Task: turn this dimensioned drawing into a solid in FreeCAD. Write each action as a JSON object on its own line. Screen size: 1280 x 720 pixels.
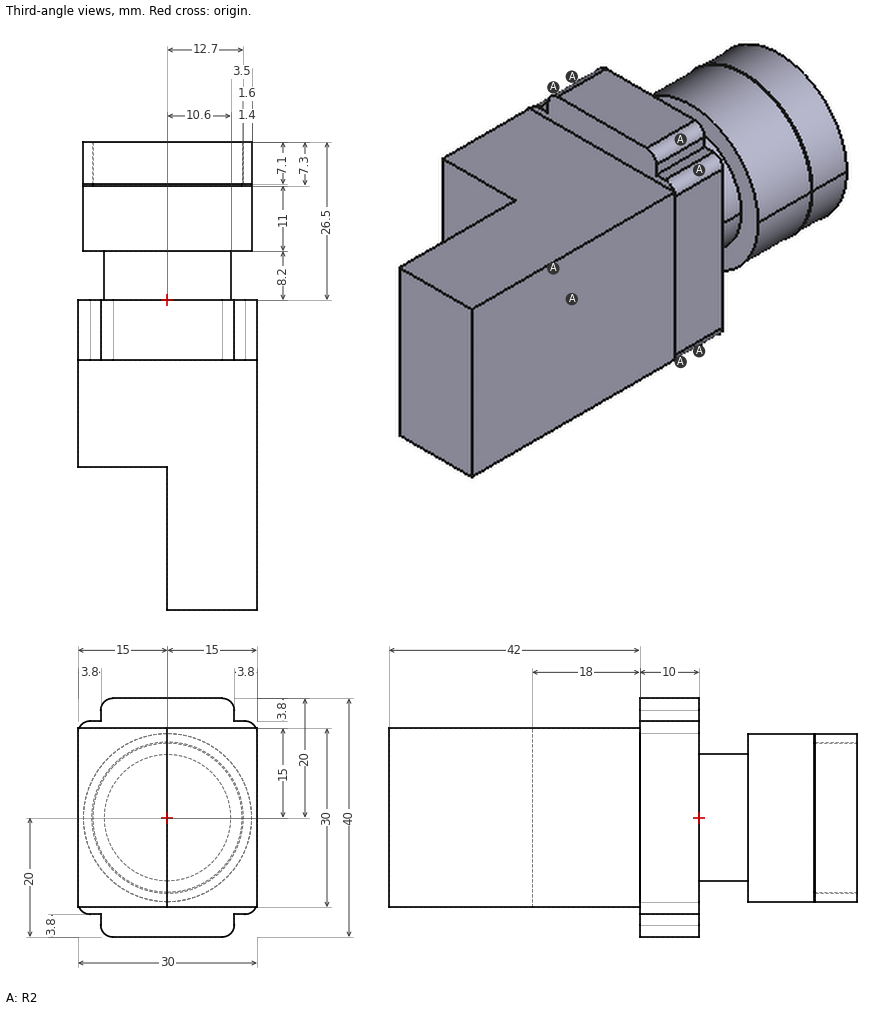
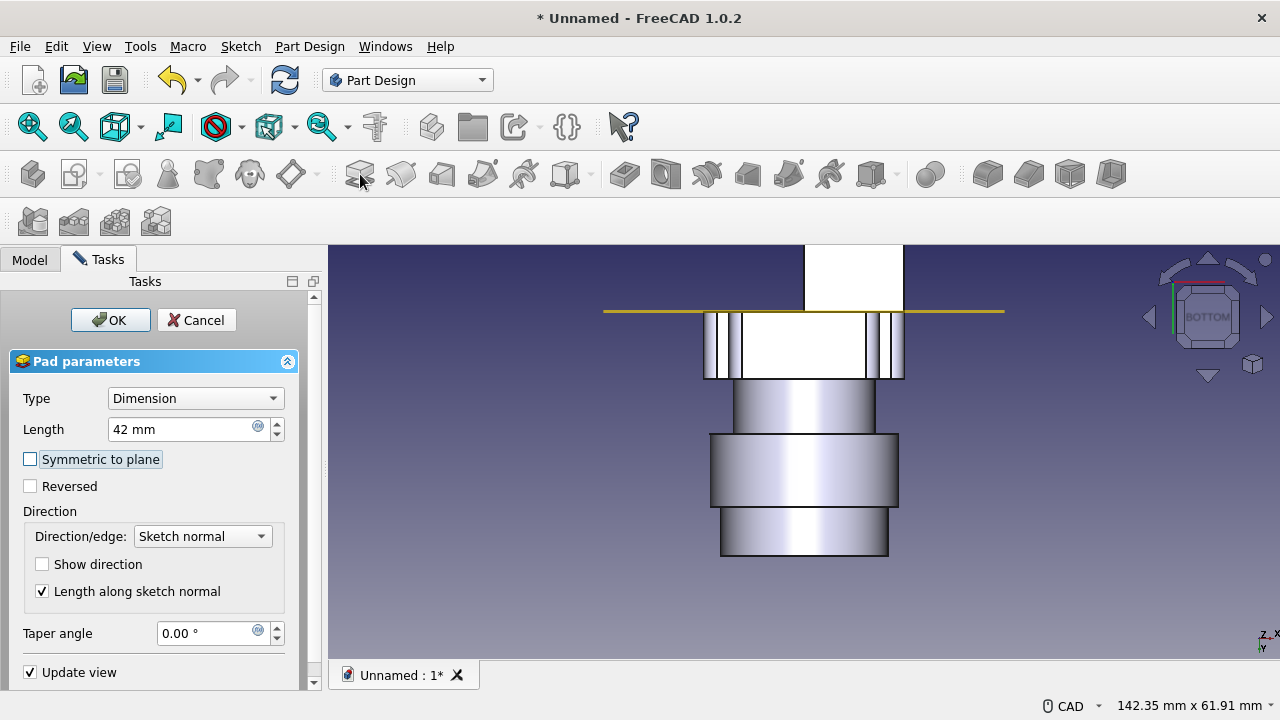
{"action": "left_click", "coordinate": [111, 320]}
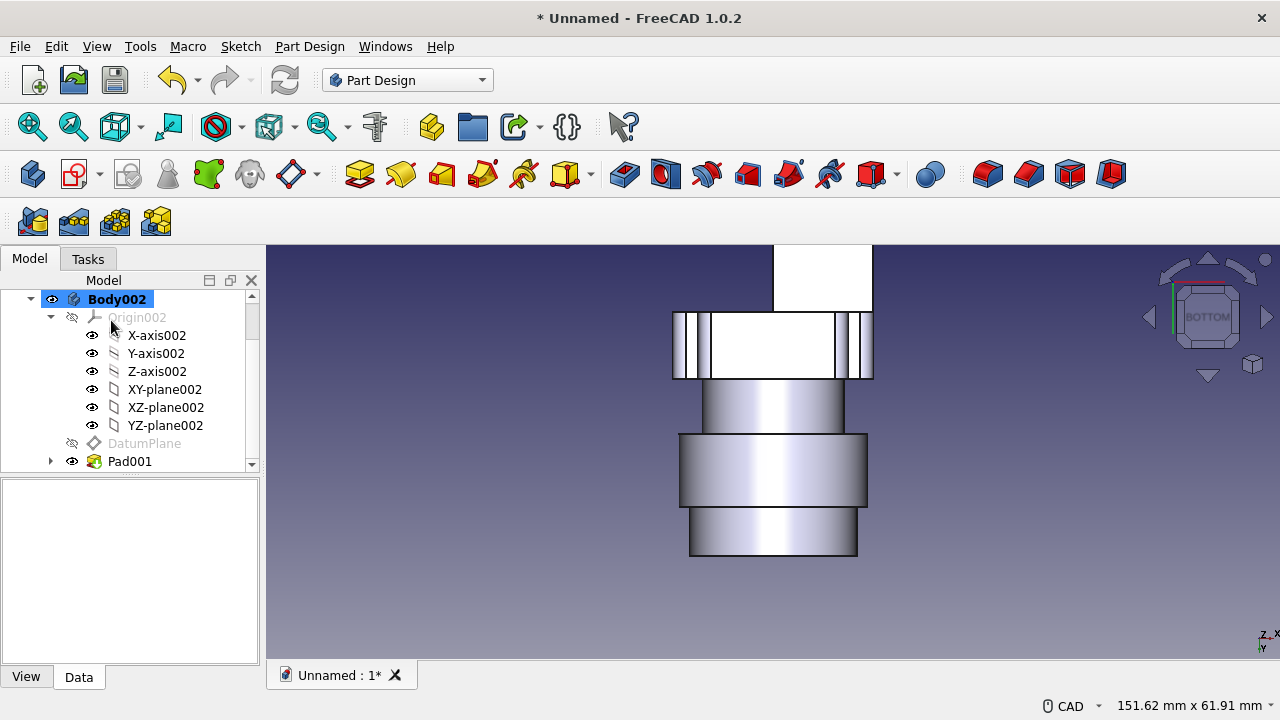
{"action": "key", "text": "v f"}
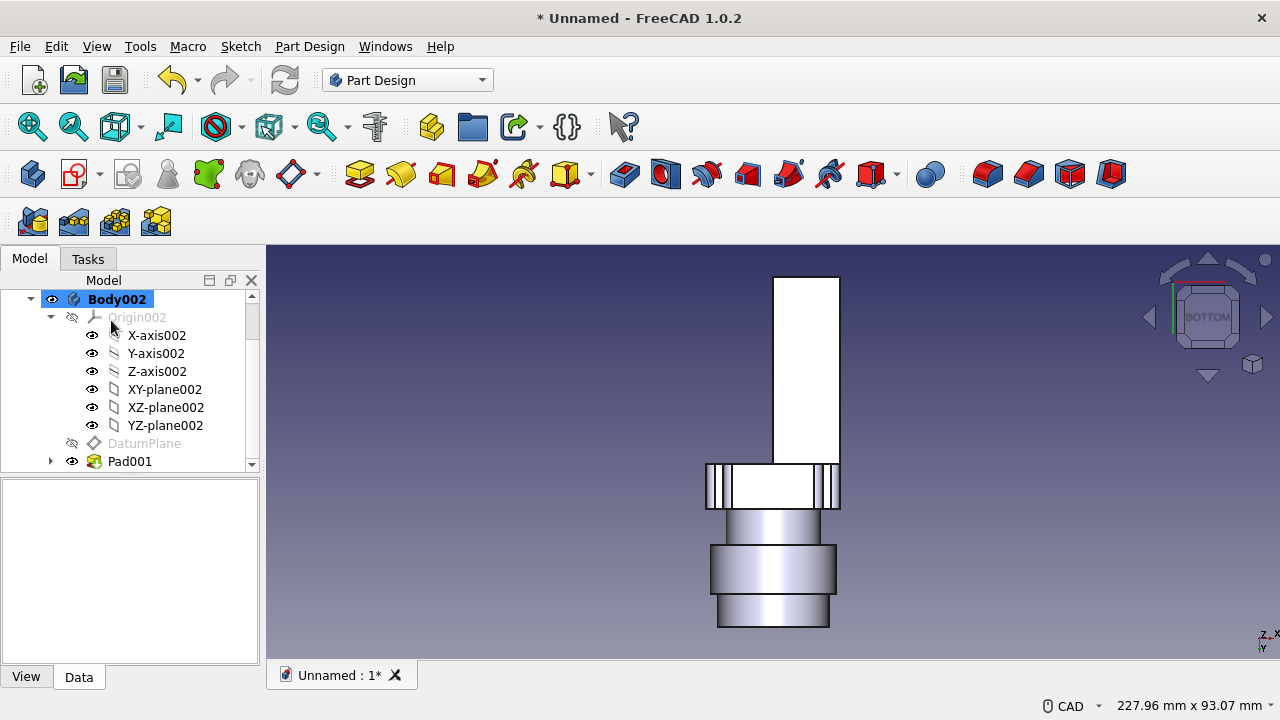
{"action": "key", "text": "4"}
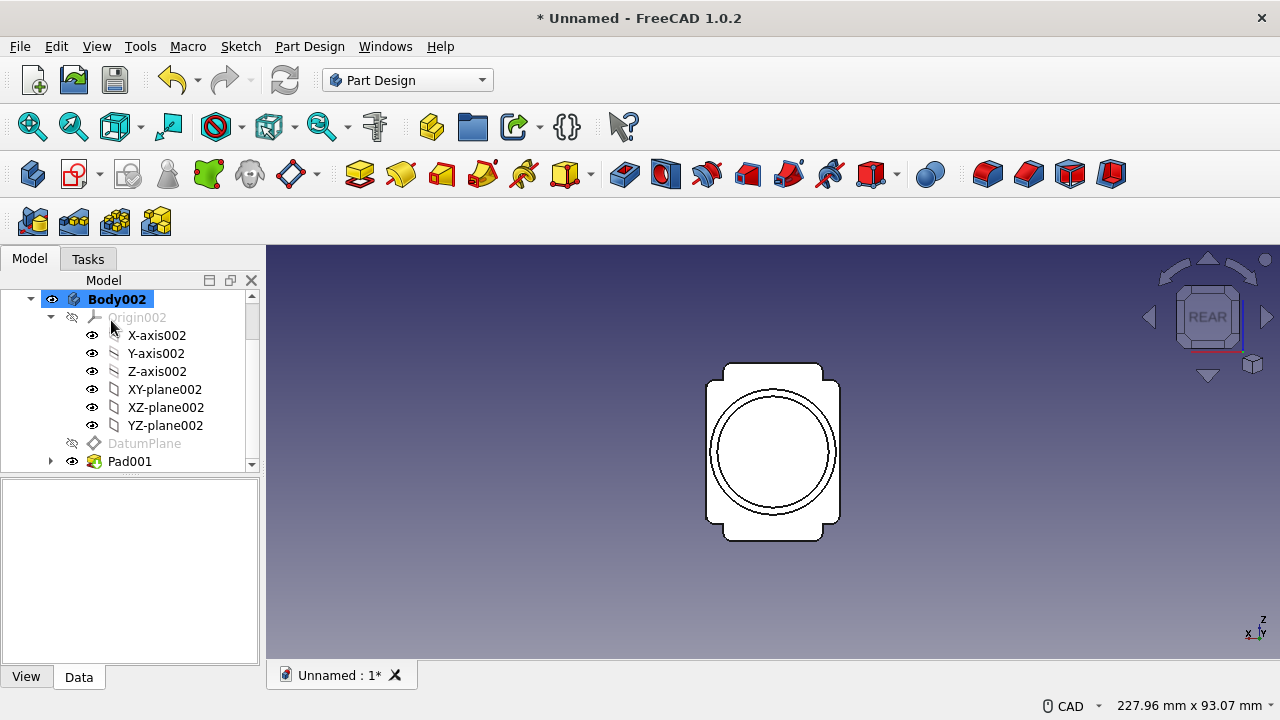
{"action": "key", "text": "v f"}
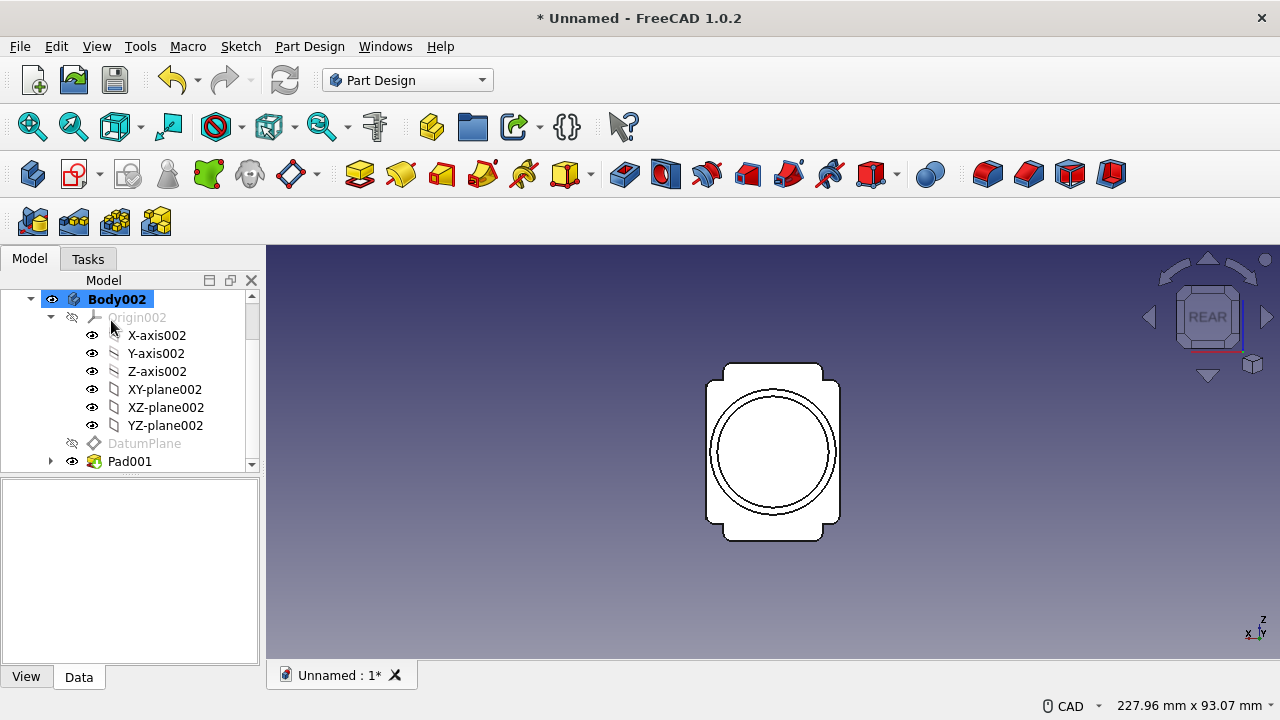
{"action": "key", "text": "5"}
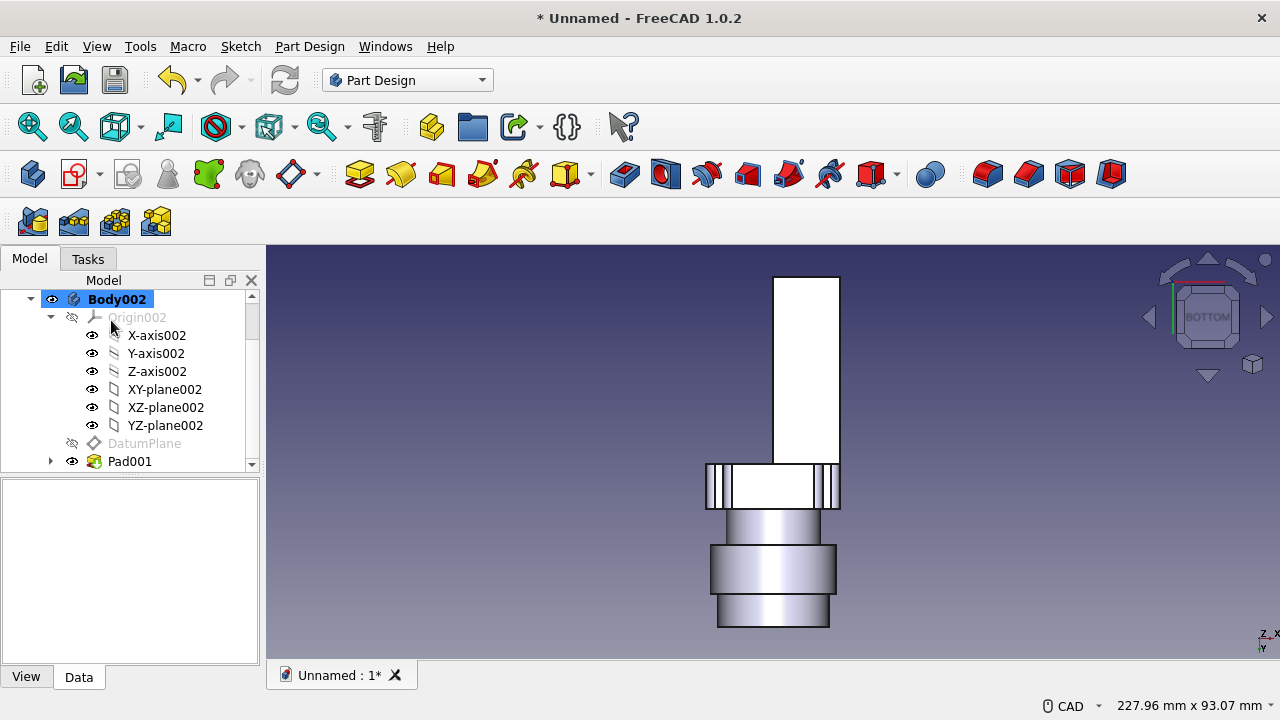
{"action": "key", "text": "3"}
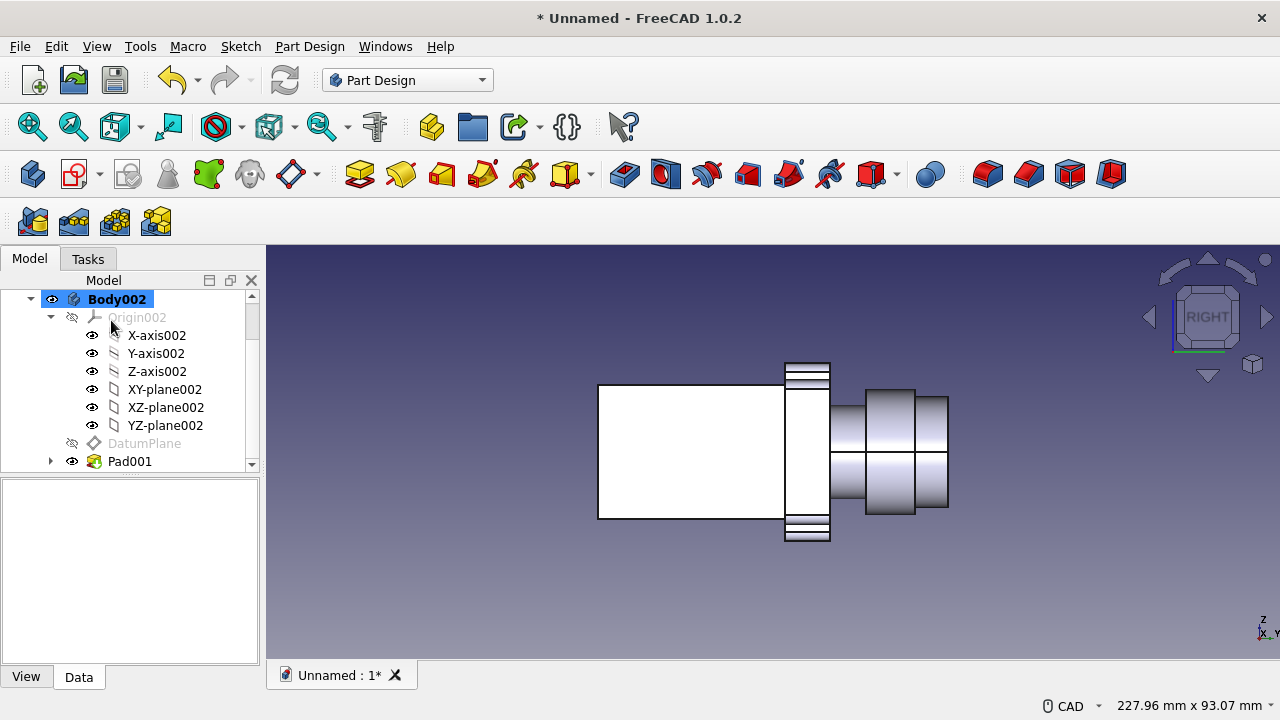
{"action": "key", "text": "v f"}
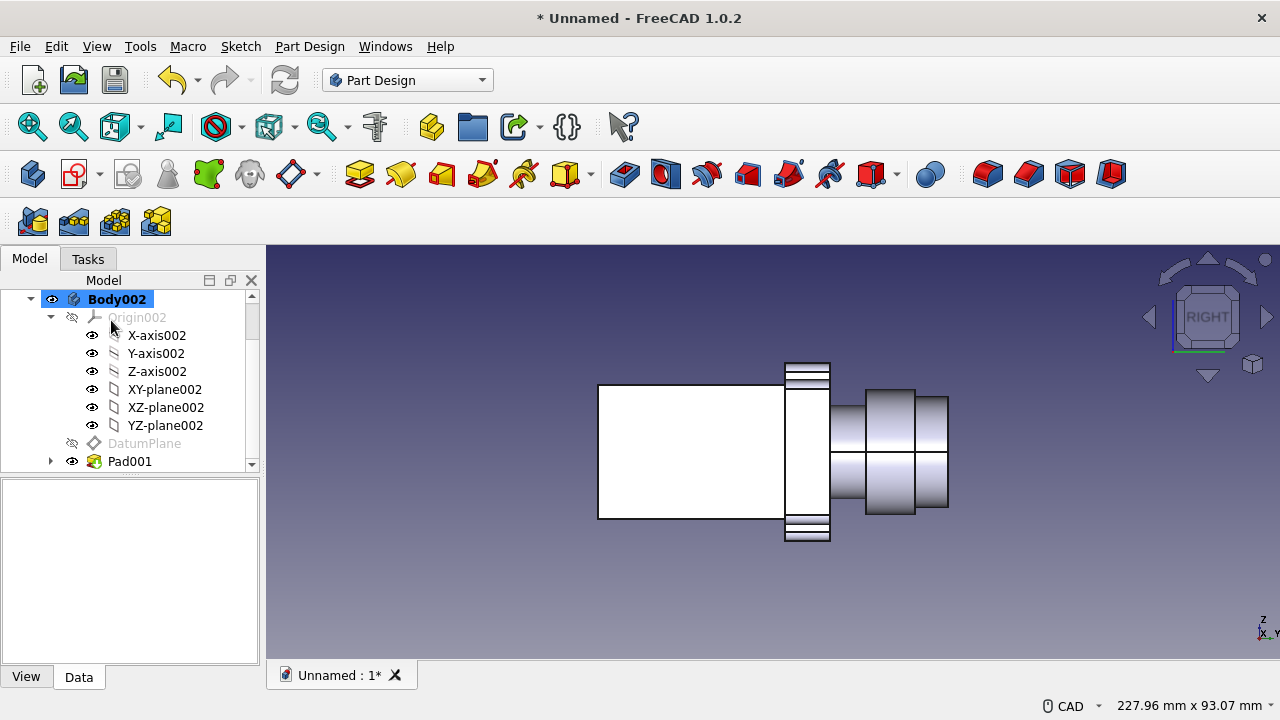
{"action": "left_click", "coordinate": [137, 407]}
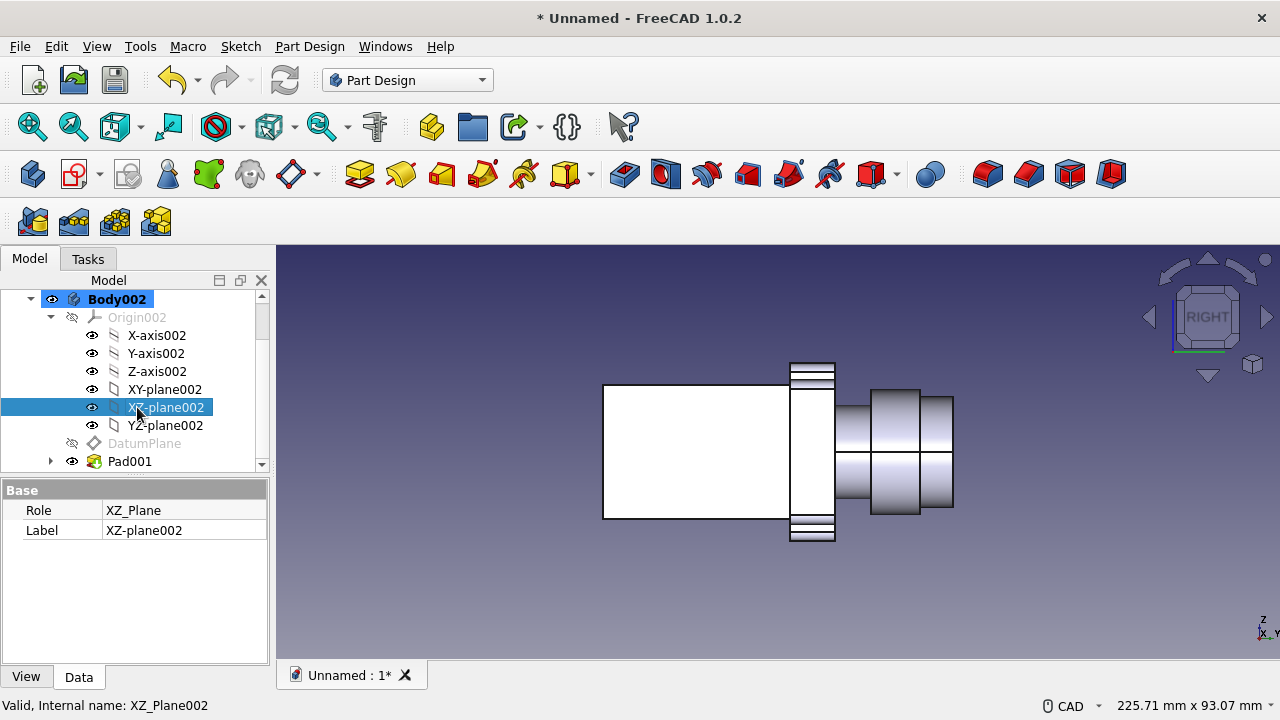
{"action": "left_click", "coordinate": [290, 174]}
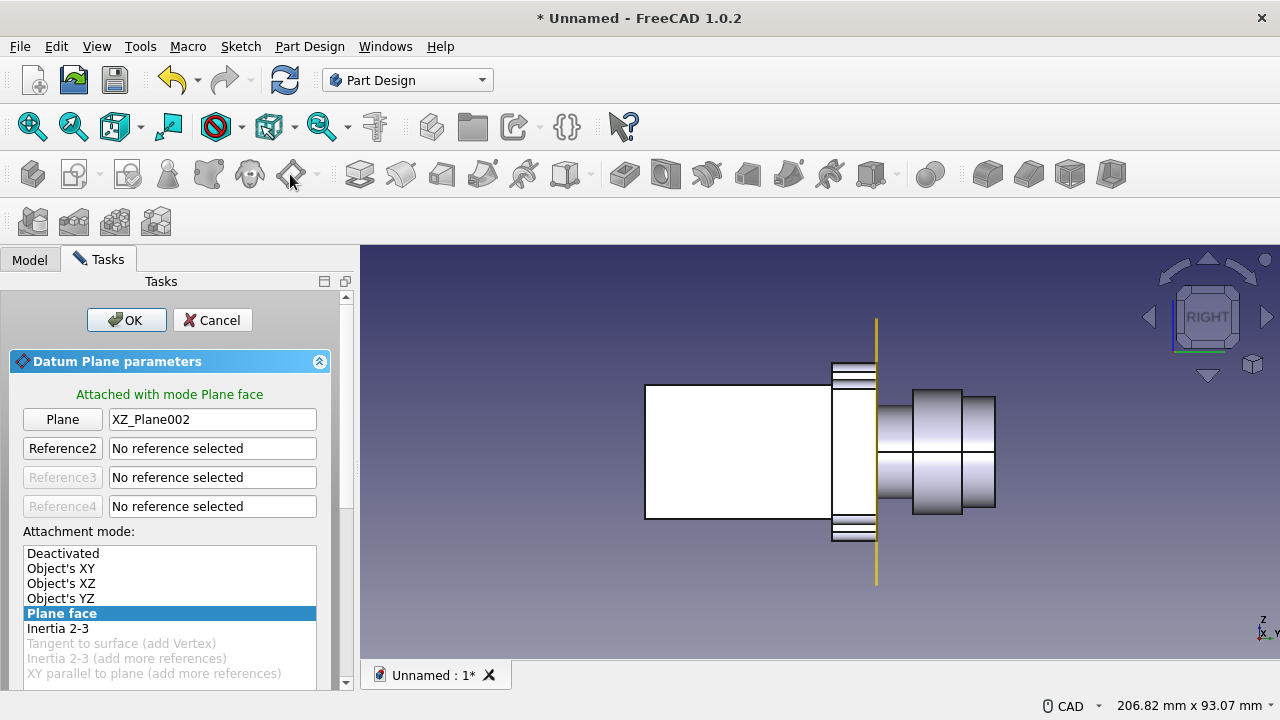
{"action": "scroll", "coordinate": [346, 490], "scroll_direction": "down", "scroll_amount": 4}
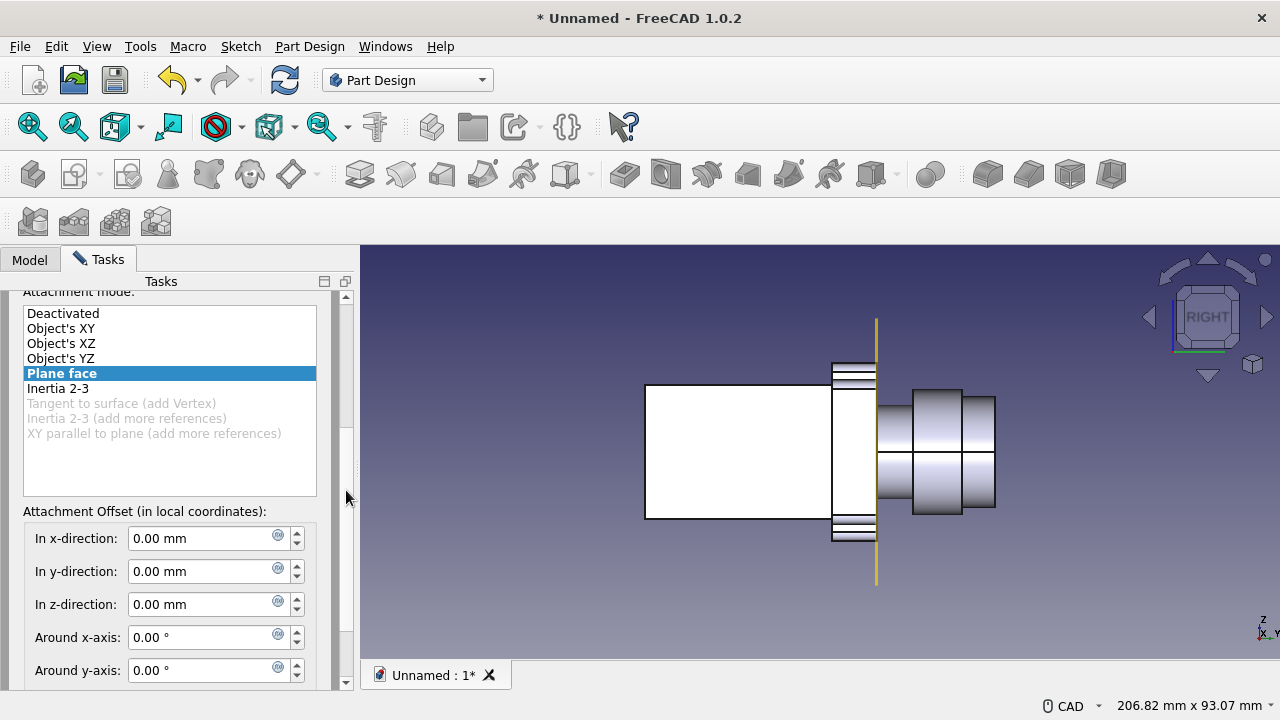
{"action": "triple_click", "coordinate": [210, 604]}